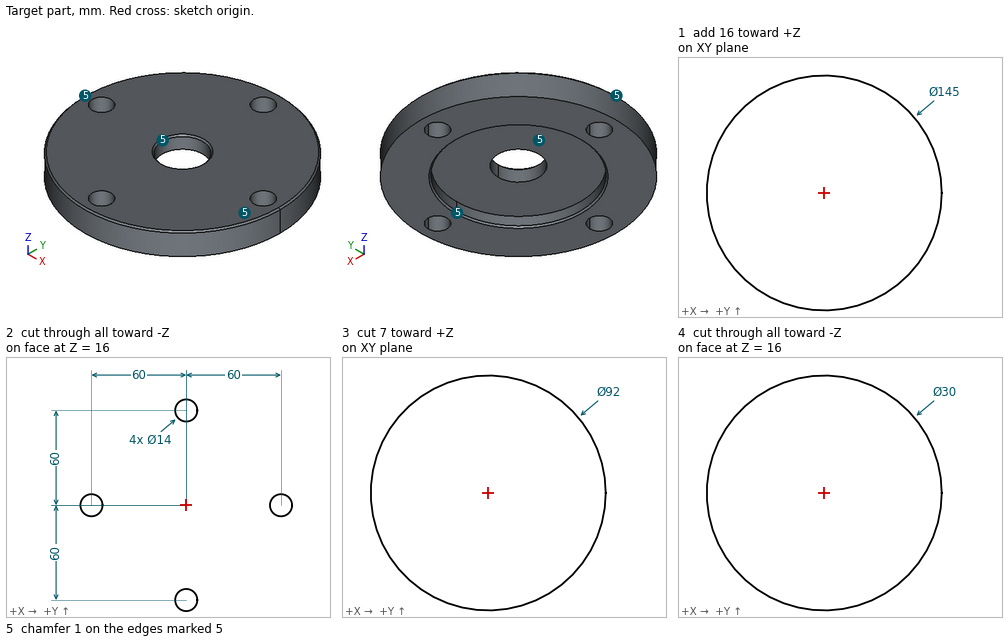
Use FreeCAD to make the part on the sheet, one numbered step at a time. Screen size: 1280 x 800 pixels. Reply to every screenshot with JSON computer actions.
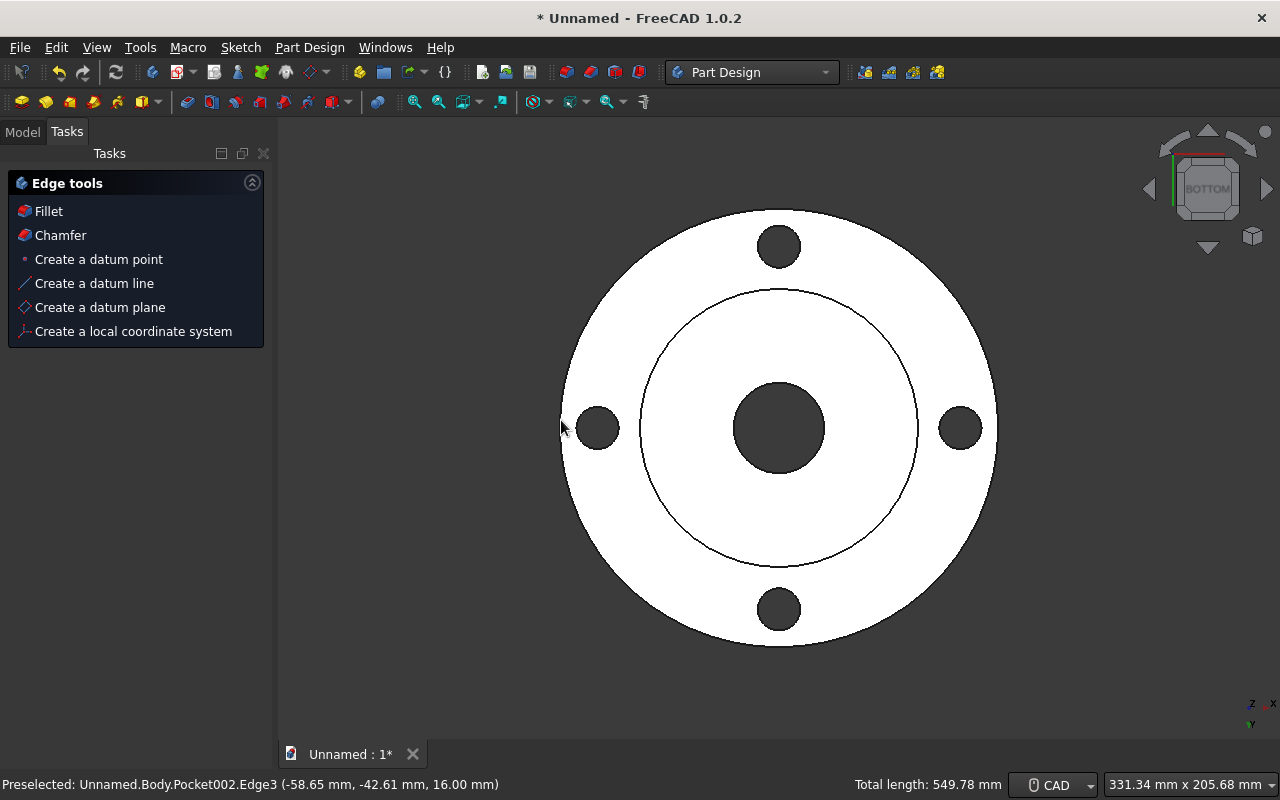
{"action": "left_click", "coordinate": [640, 427], "text": "ctrl"}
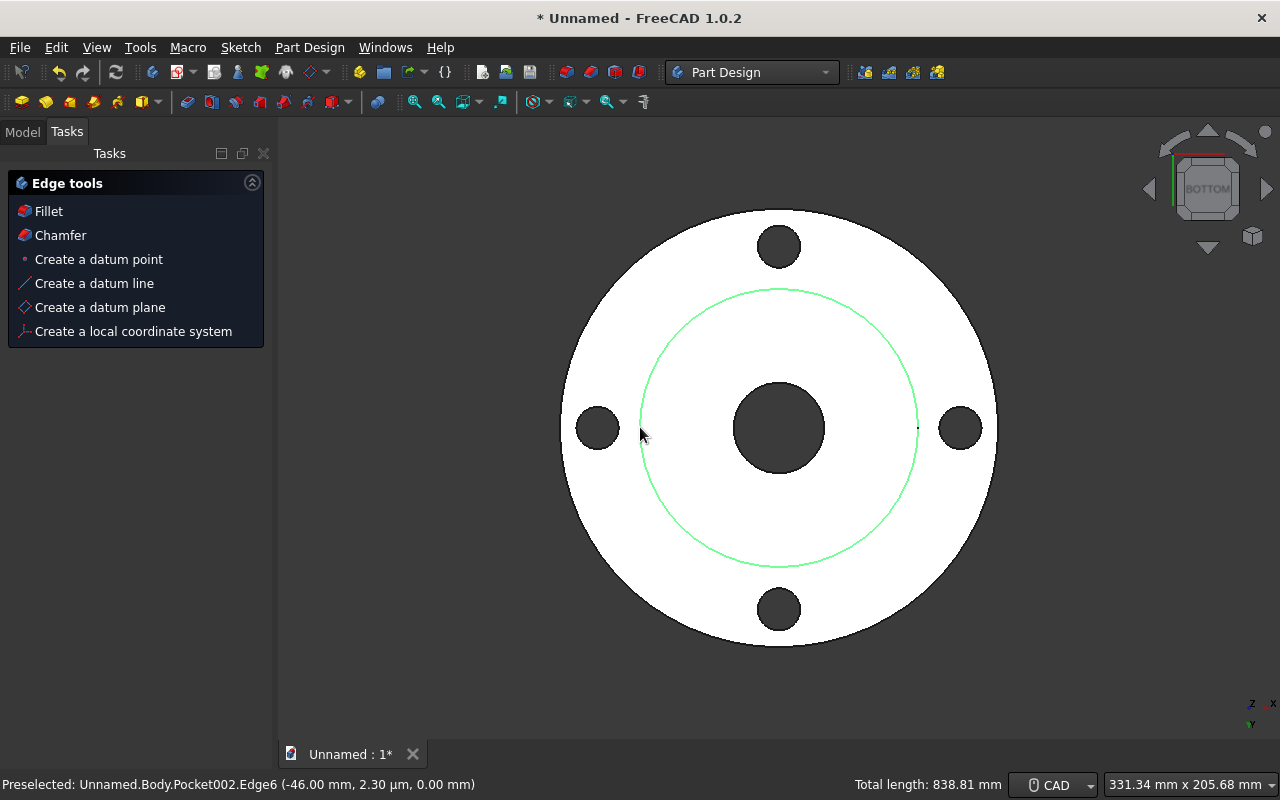
{"action": "left_click", "coordinate": [592, 72]}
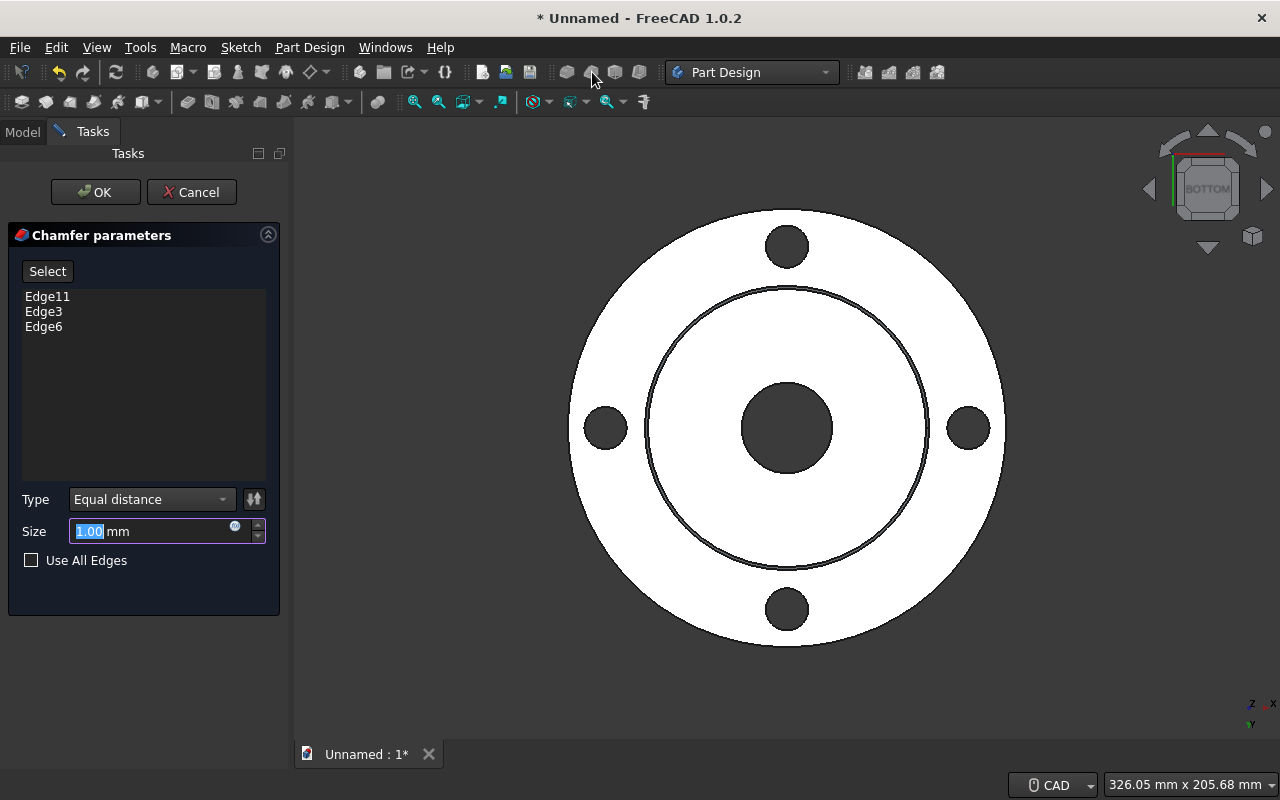
{"action": "type", "text": "1"}
{"action": "key", "text": "Tab"}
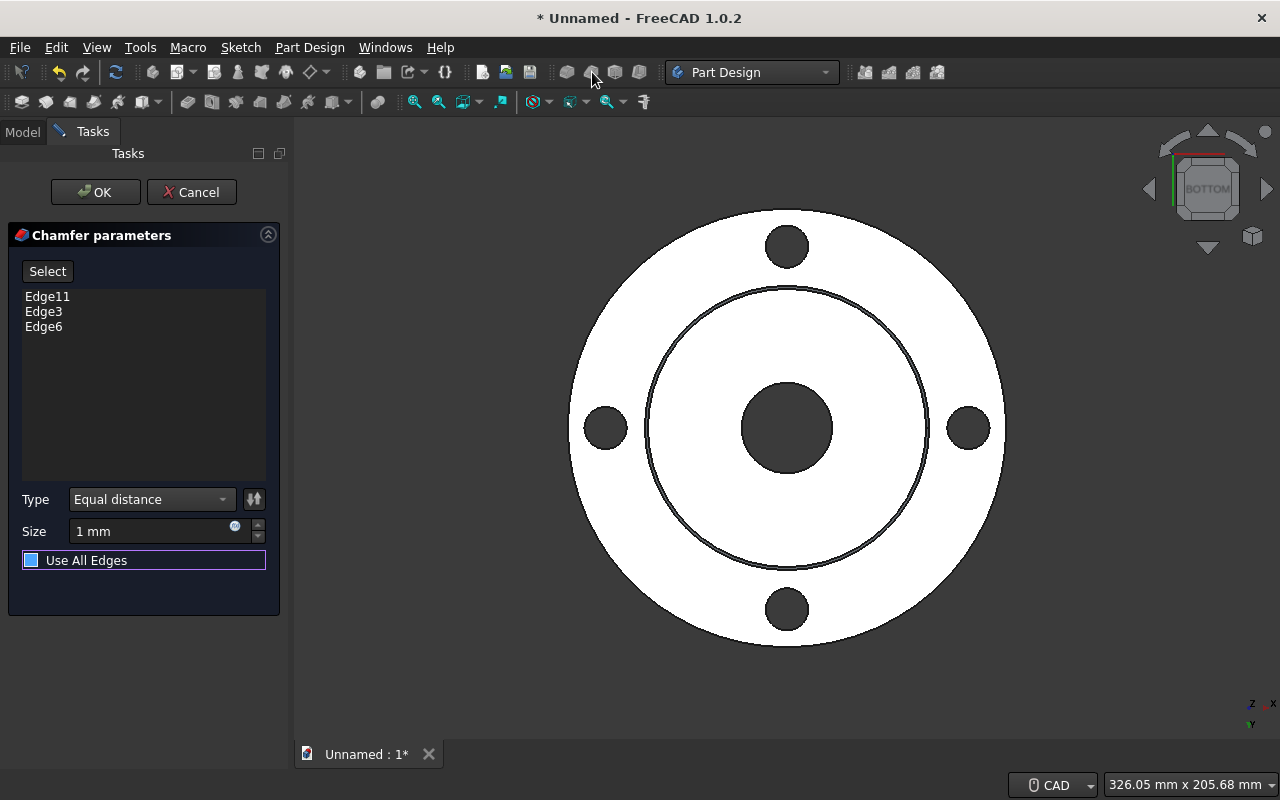
{"action": "left_click", "coordinate": [96, 192]}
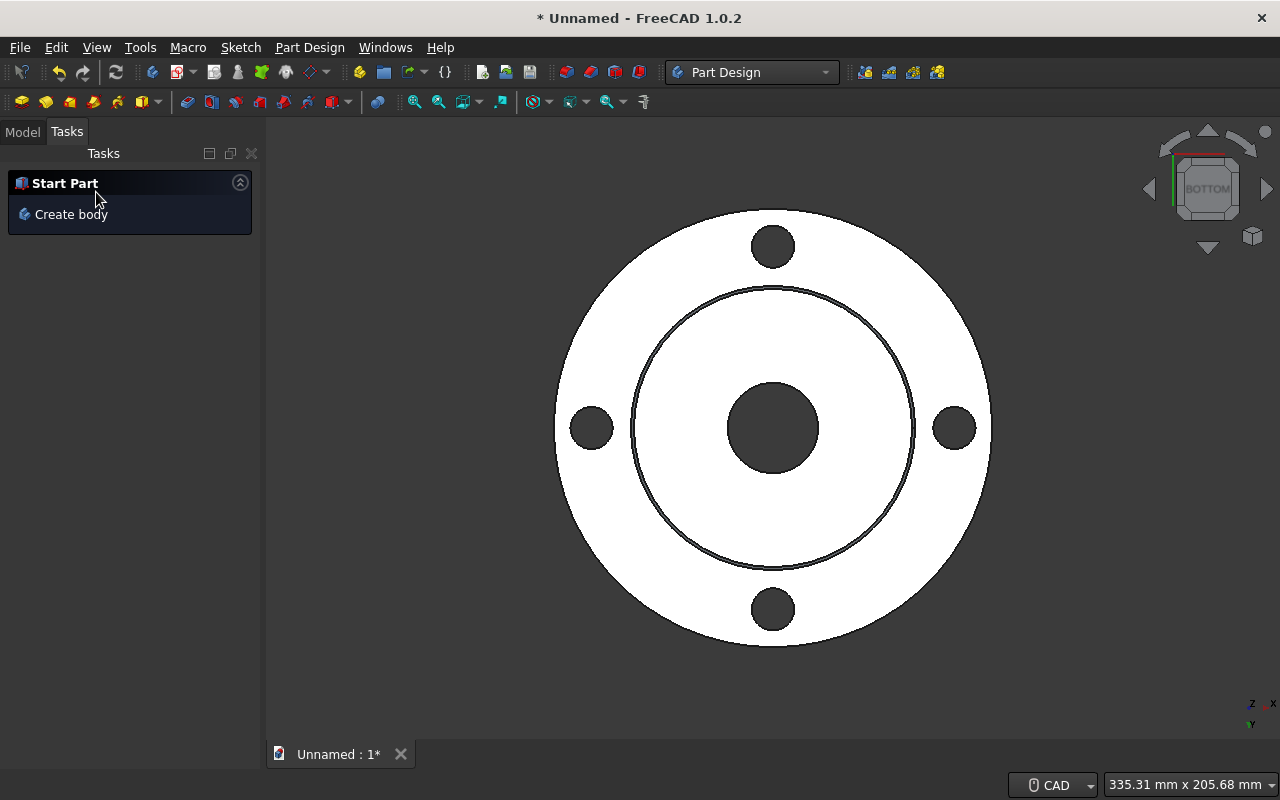
{"action": "key", "text": "0"}